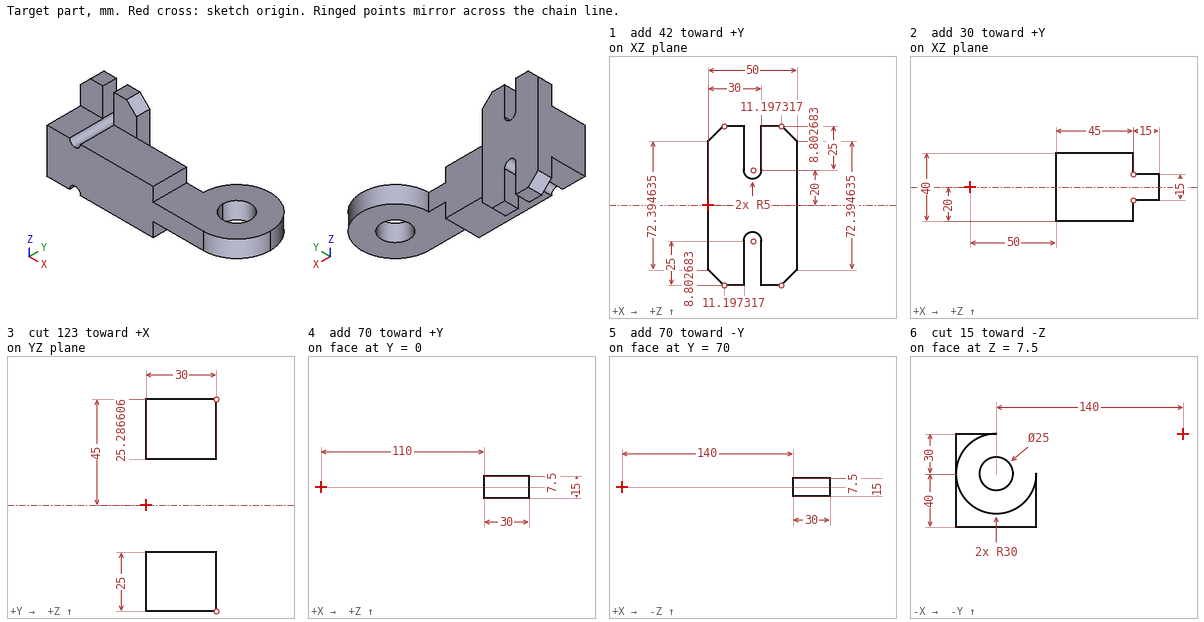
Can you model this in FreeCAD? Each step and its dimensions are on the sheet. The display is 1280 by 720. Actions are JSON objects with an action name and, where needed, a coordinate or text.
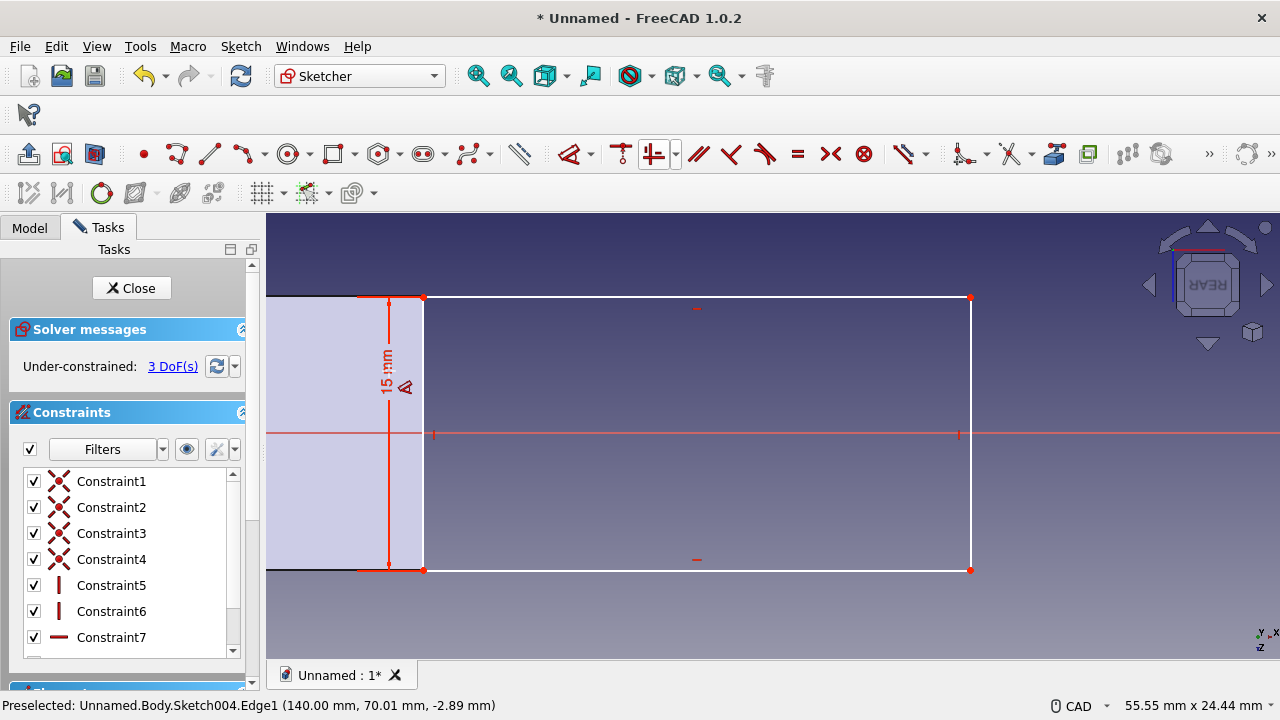
{"action": "left_click", "coordinate": [587, 571]}
{"action": "left_click", "coordinate": [697, 605]}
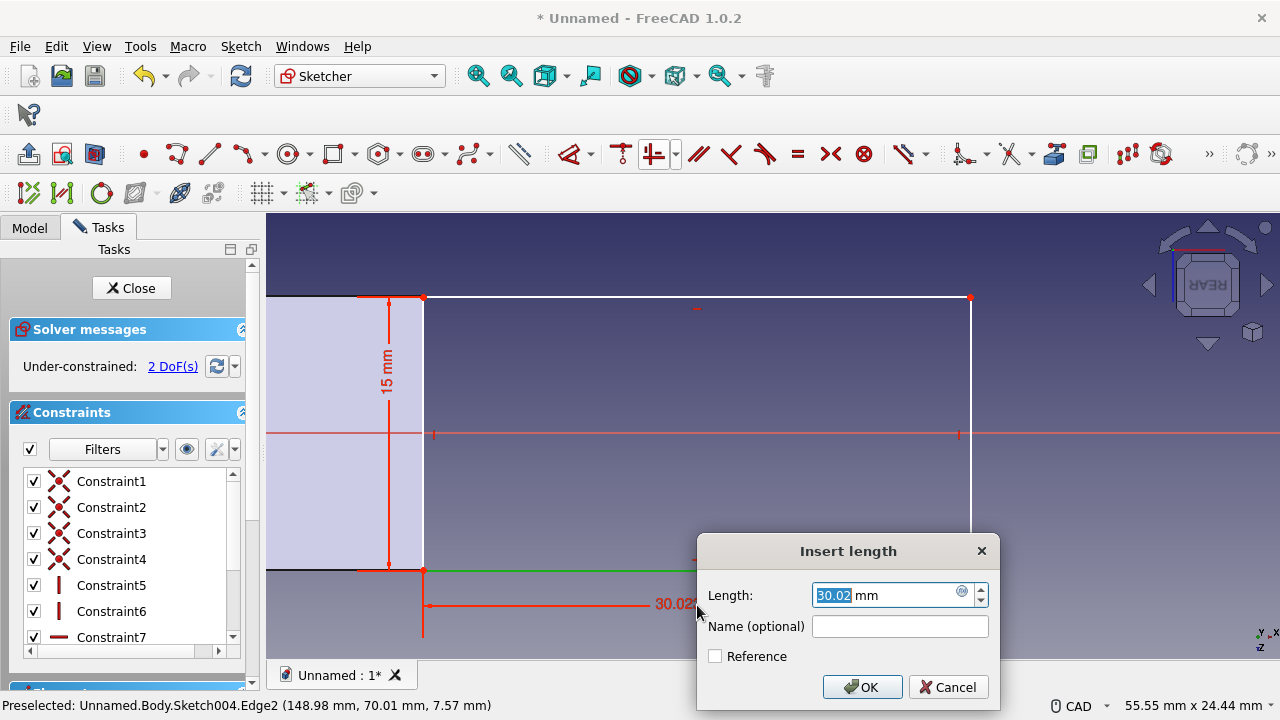
{"action": "type", "text": "30"}
{"action": "key", "text": "Return"}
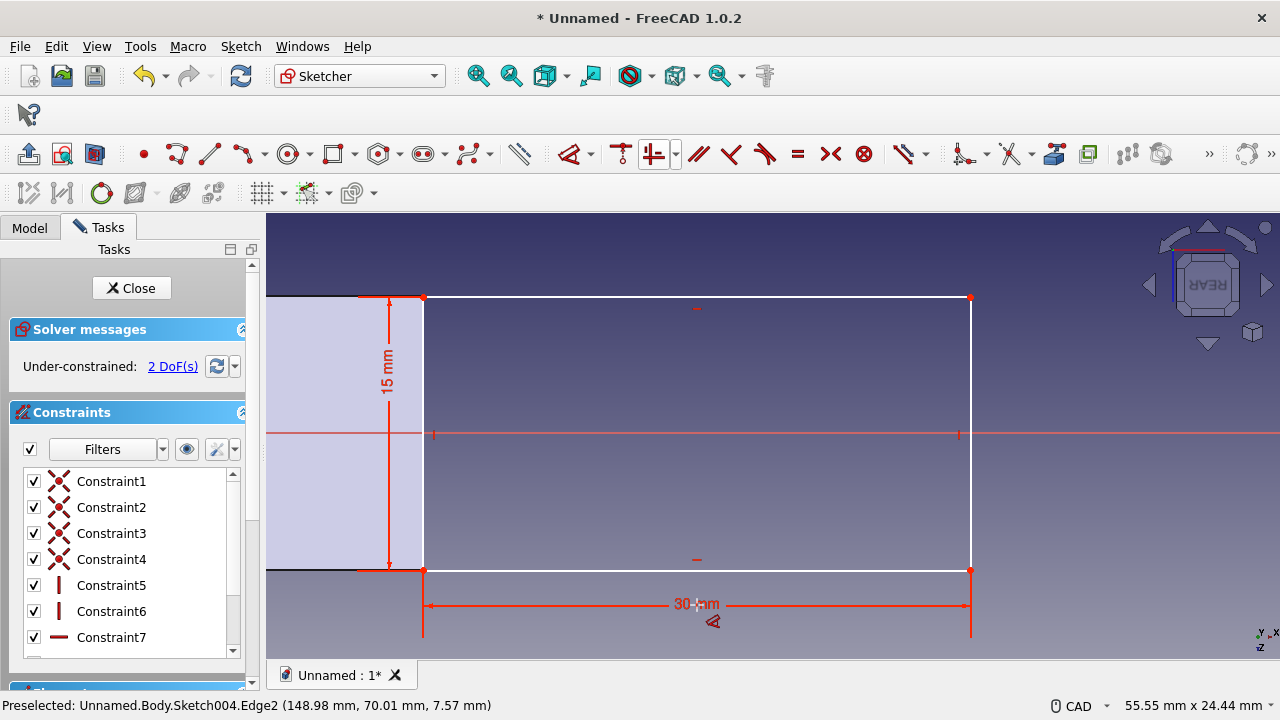
{"action": "left_click", "coordinate": [423, 297]}
{"action": "left_click", "coordinate": [359, 263]}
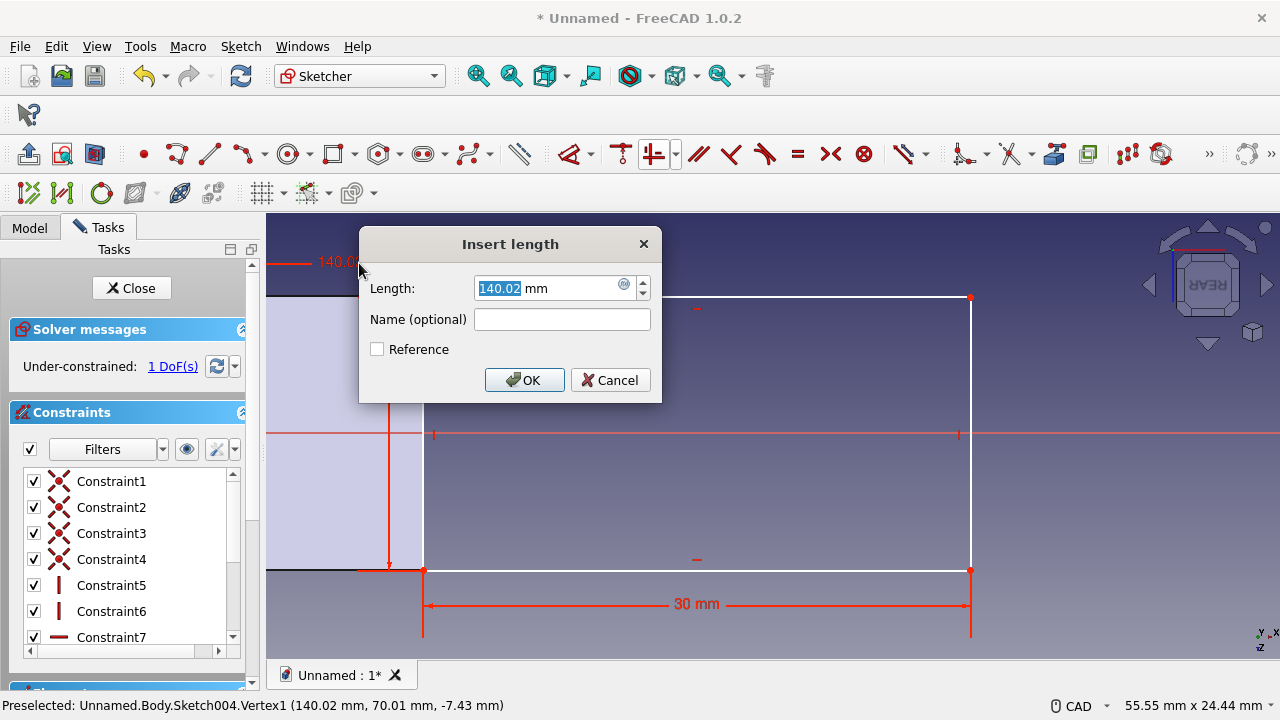
{"action": "type", "text": "140"}
{"action": "key", "text": "Return"}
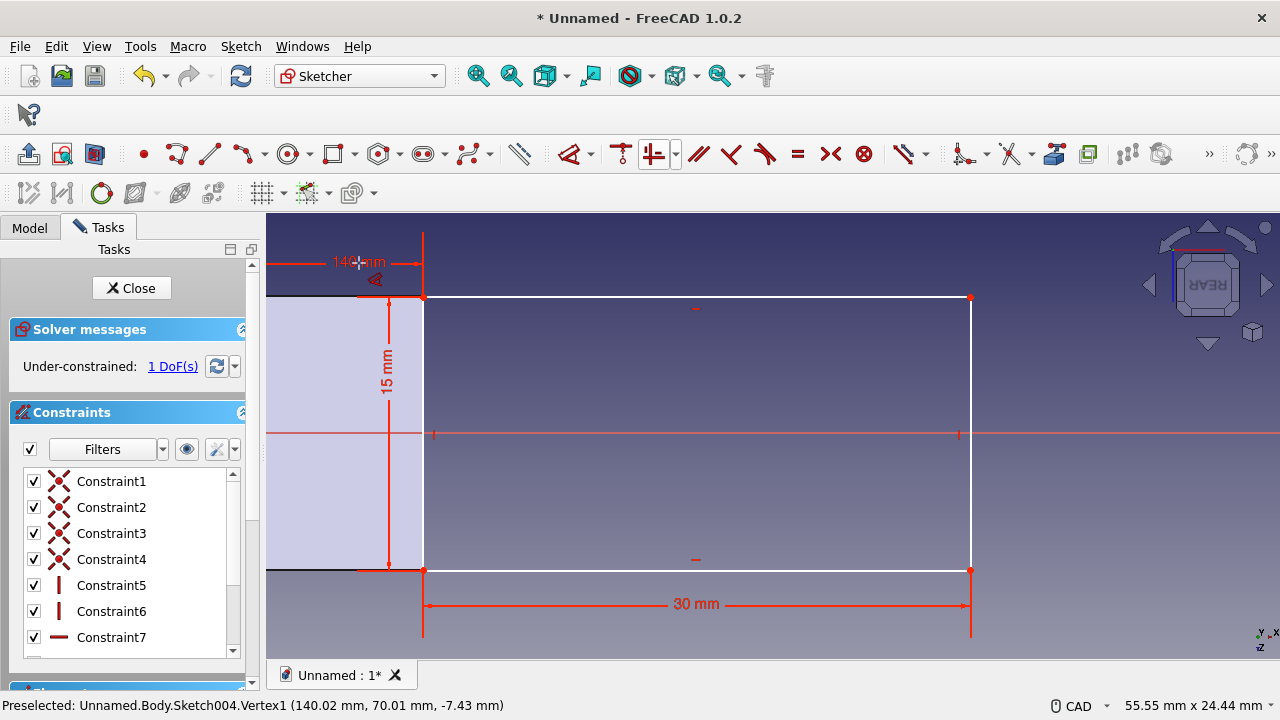
{"action": "left_click", "coordinate": [423, 297]}
{"action": "left_click", "coordinate": [457, 334]}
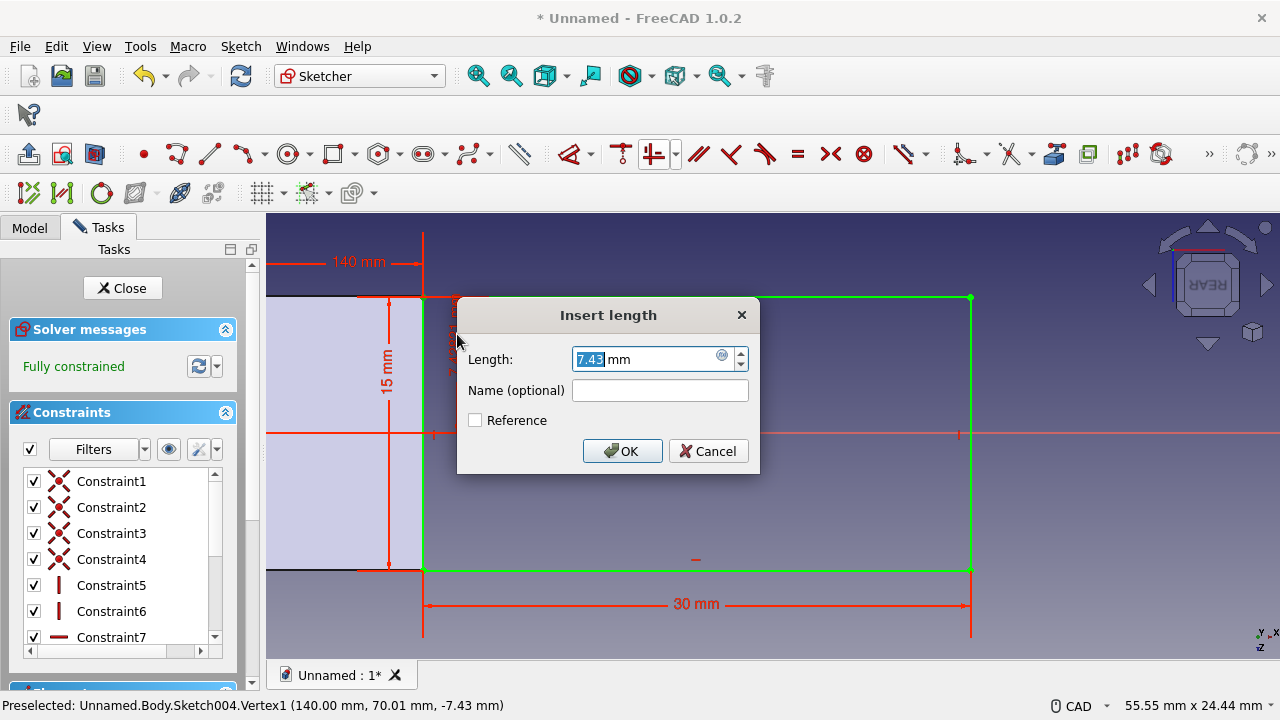
{"action": "type", "text": "7.5"}
{"action": "key", "text": "Return"}
{"action": "key", "text": "Escape"}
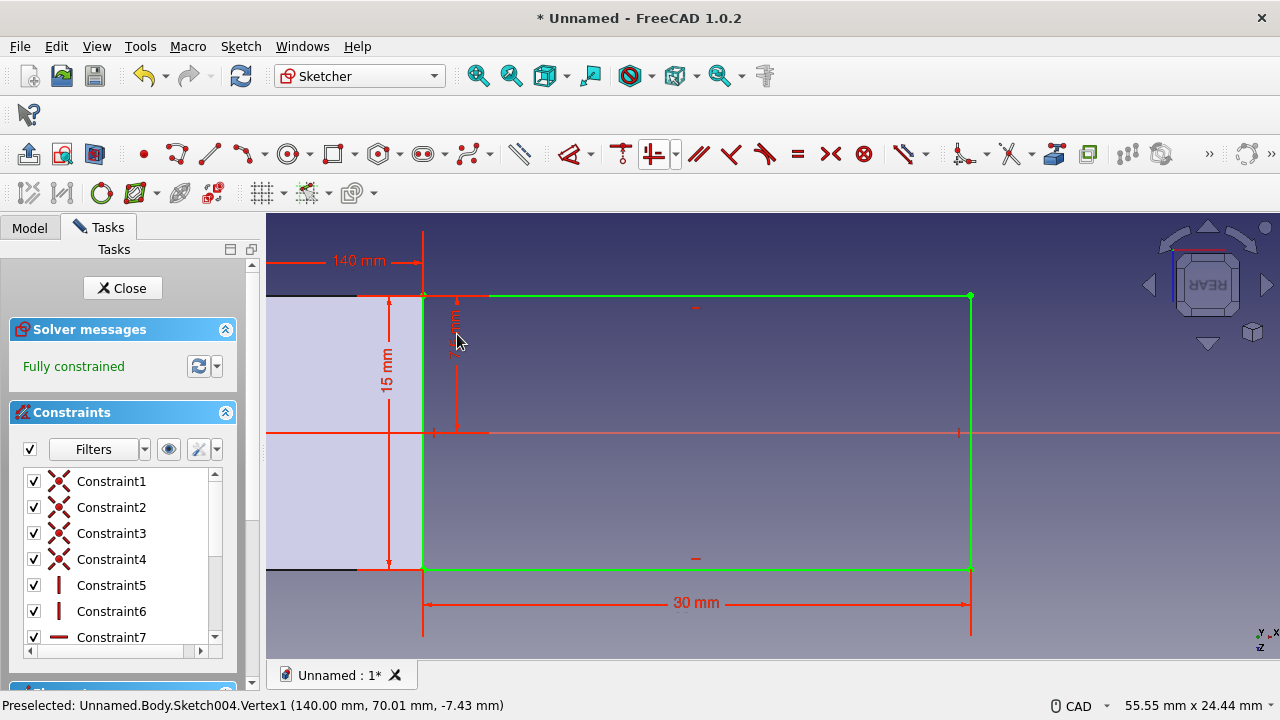
{"action": "left_click", "coordinate": [123, 288]}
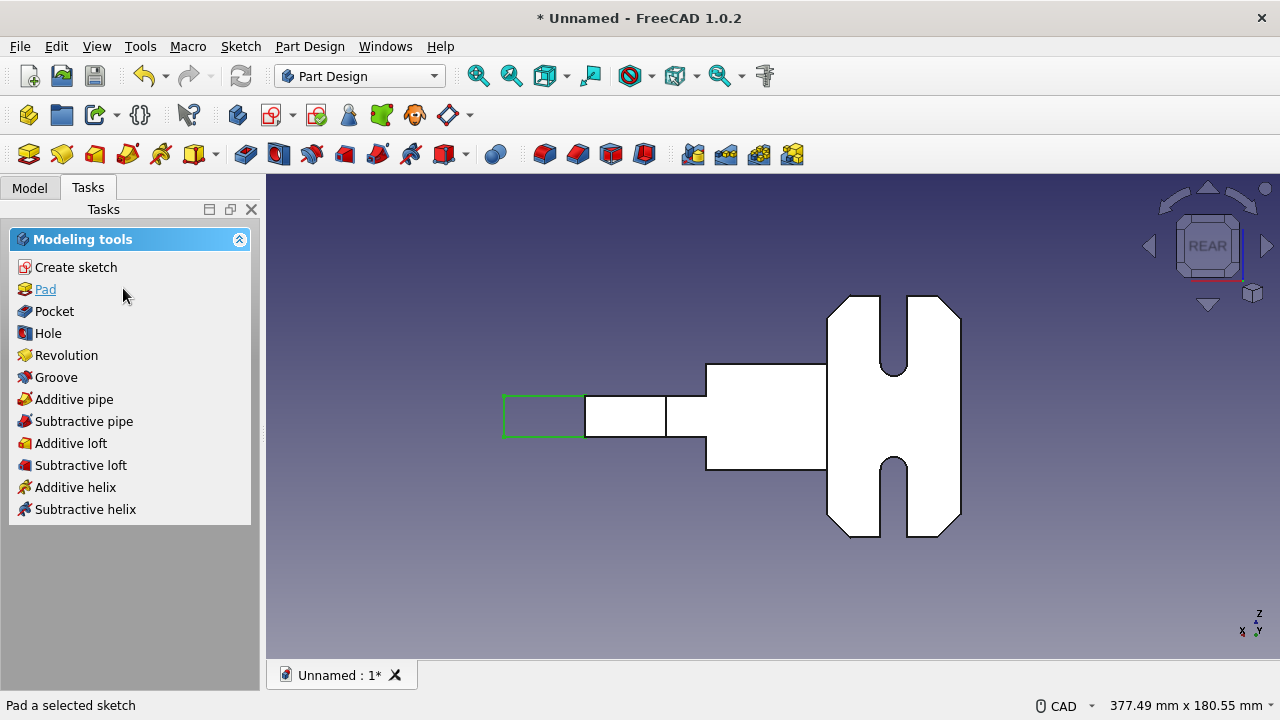
{"action": "left_click", "coordinate": [29, 154]}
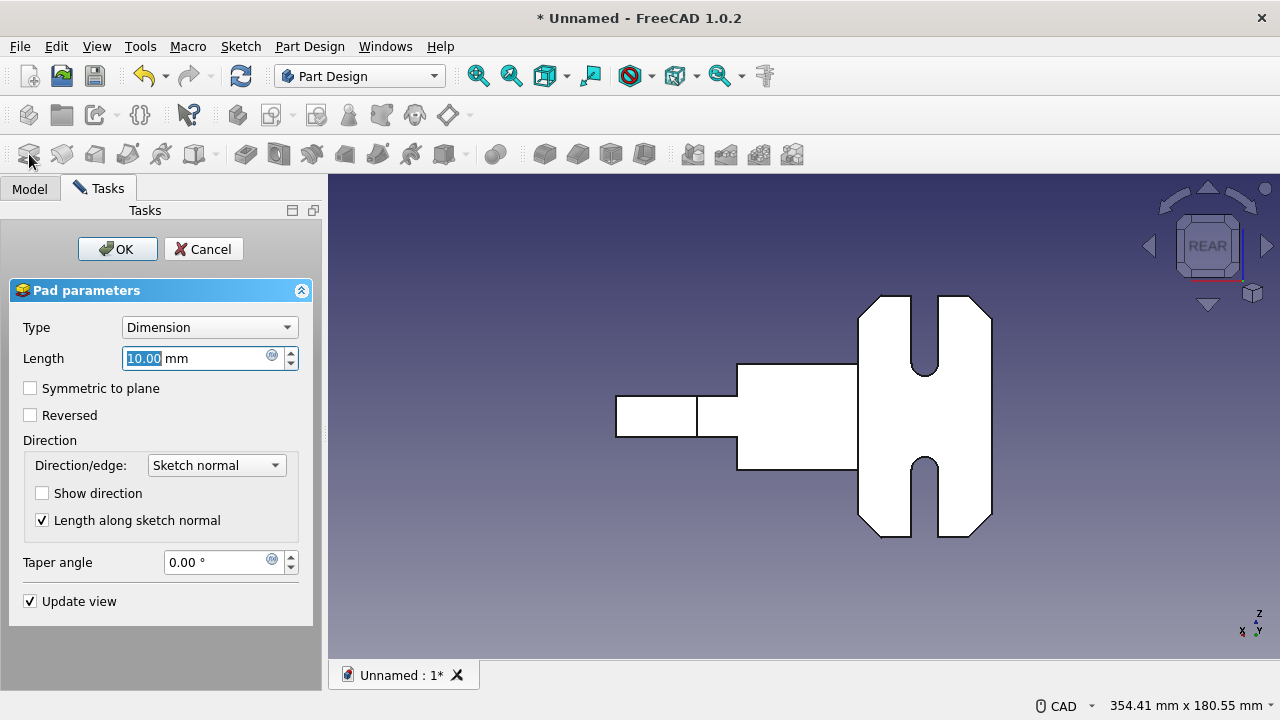
{"action": "type", "text": "70"}
{"action": "key", "text": "Tab"}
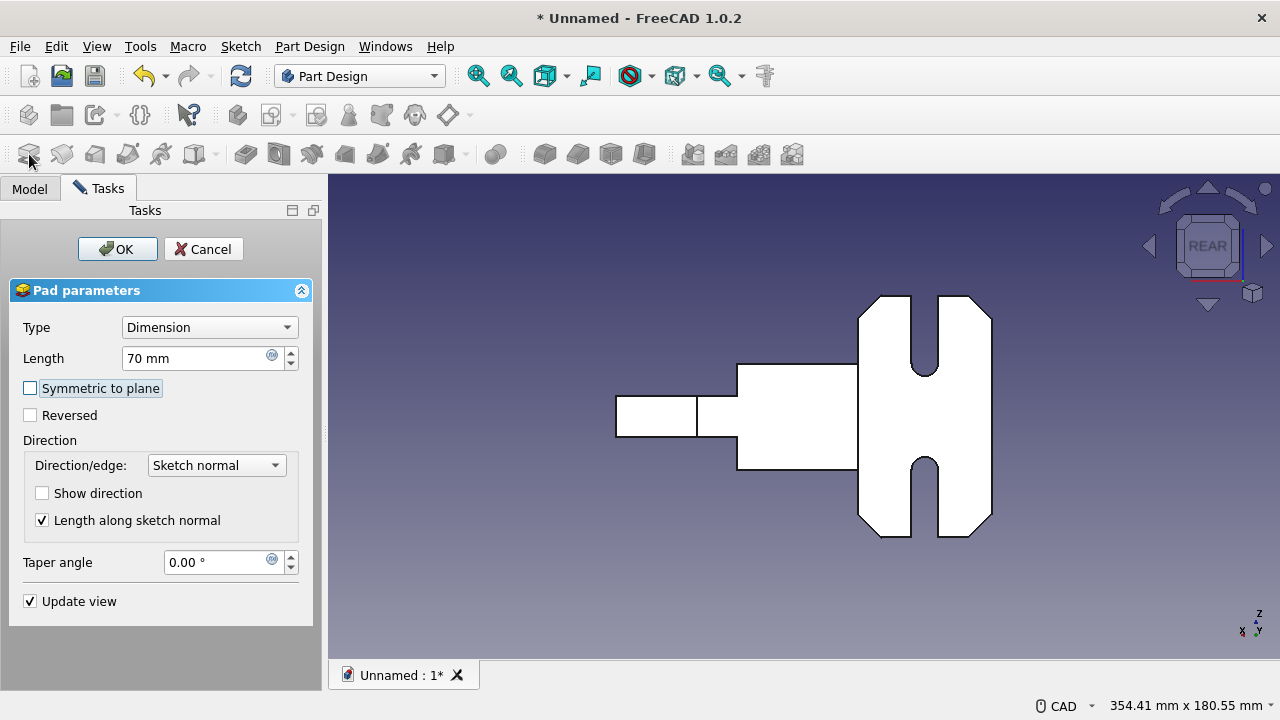
{"action": "left_click", "coordinate": [31, 415]}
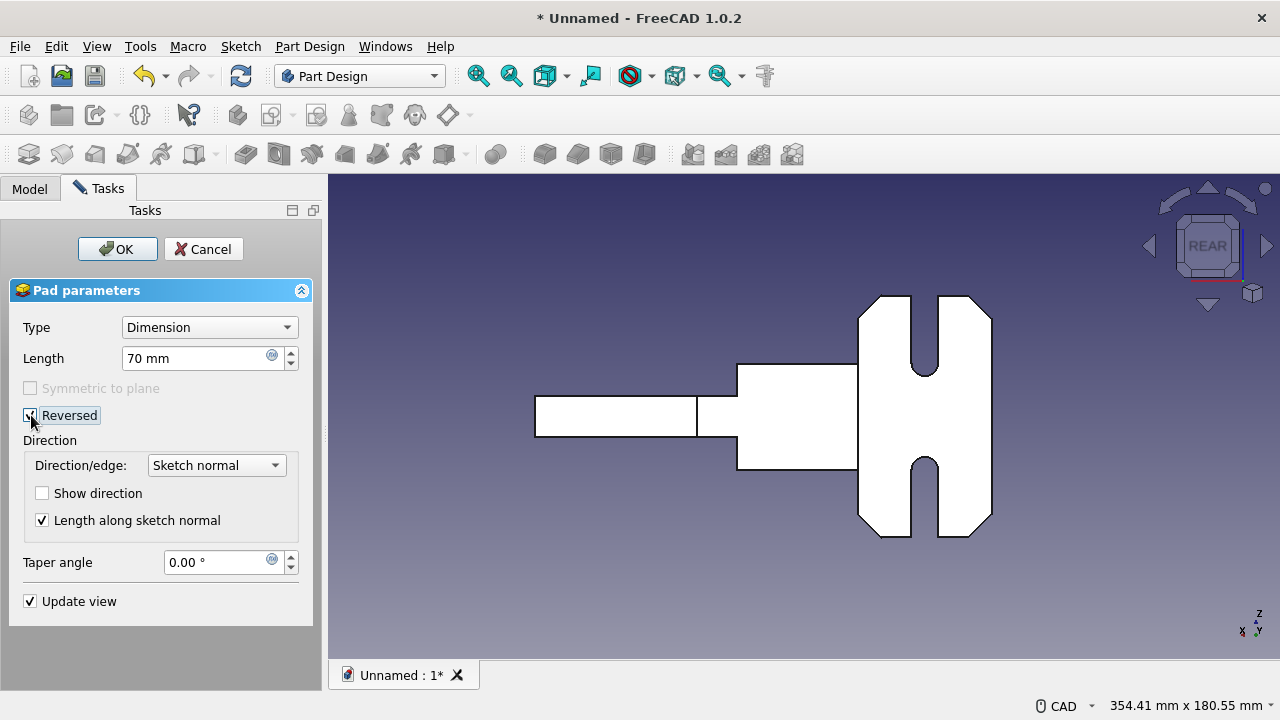
{"action": "left_click", "coordinate": [118, 249]}